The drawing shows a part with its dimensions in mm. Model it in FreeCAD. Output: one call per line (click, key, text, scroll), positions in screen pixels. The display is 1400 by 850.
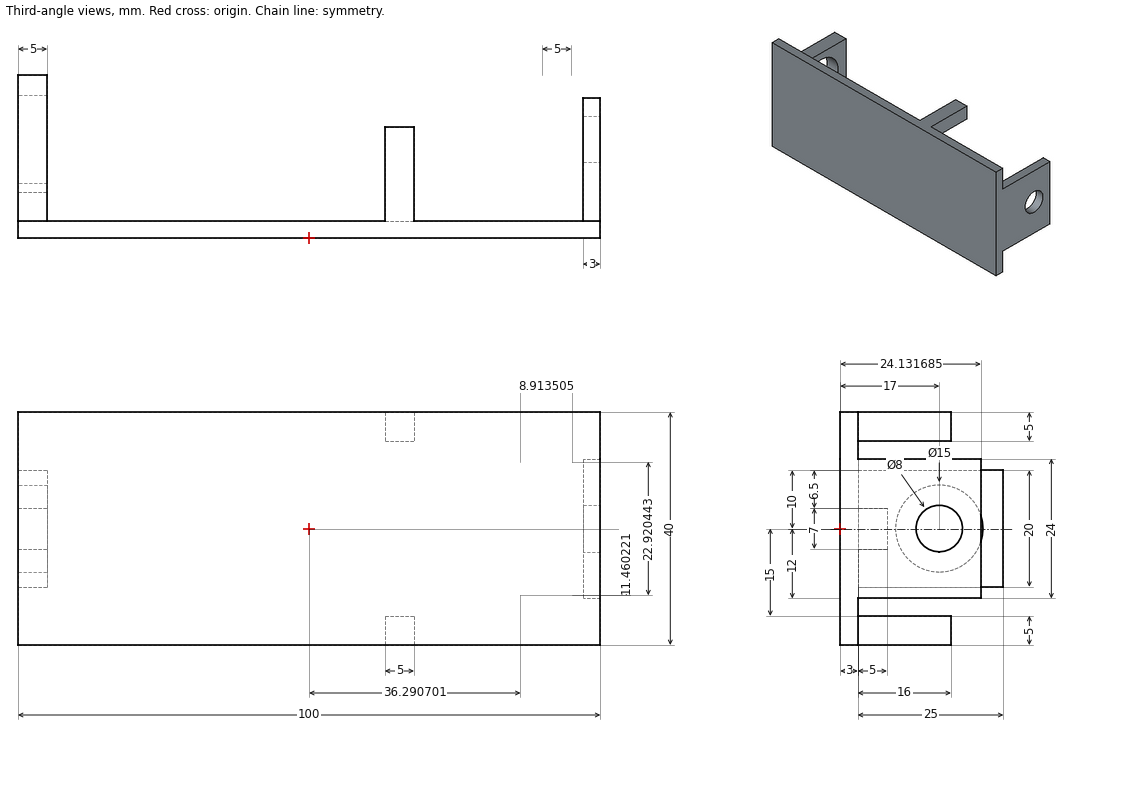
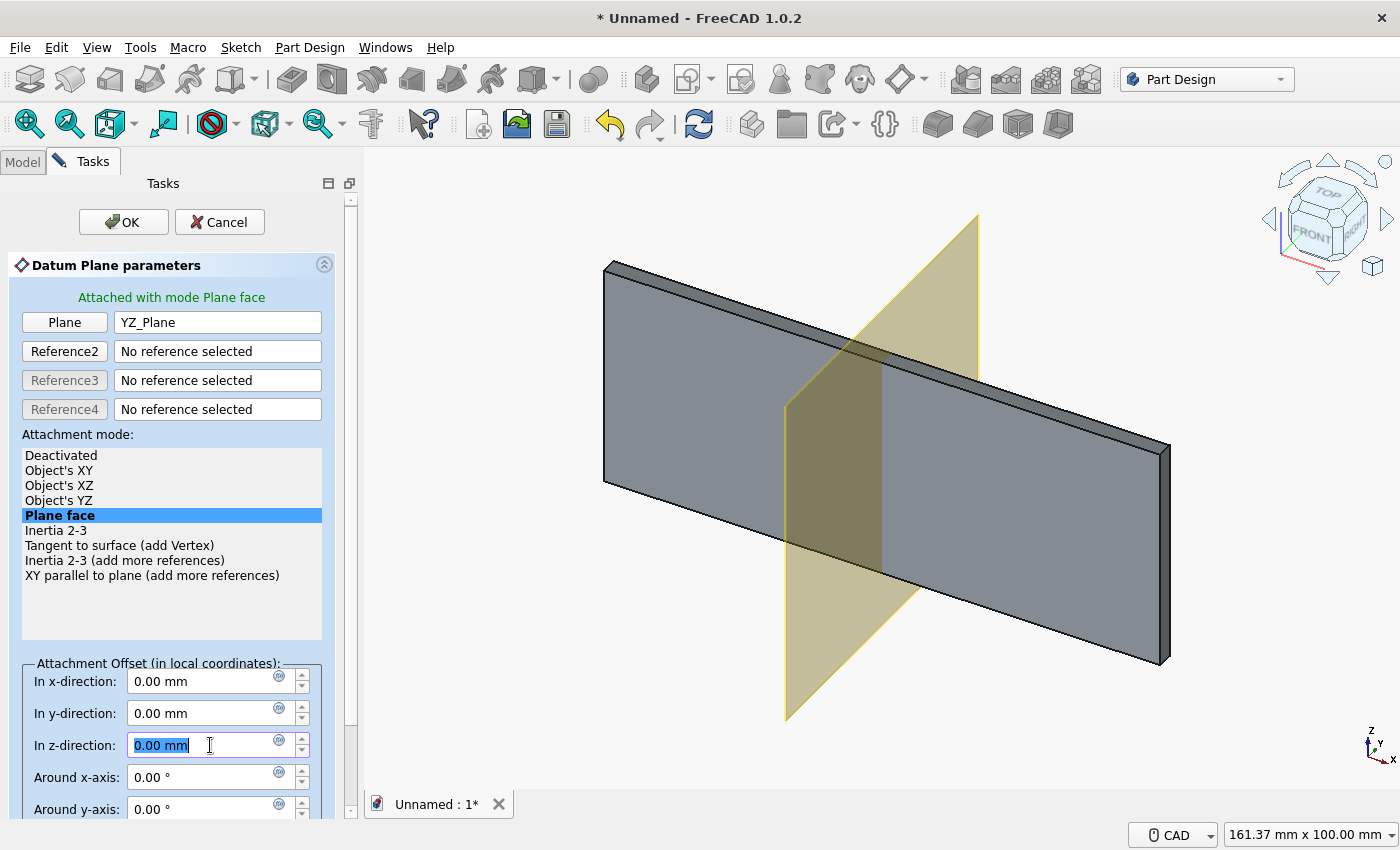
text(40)
key(Tab)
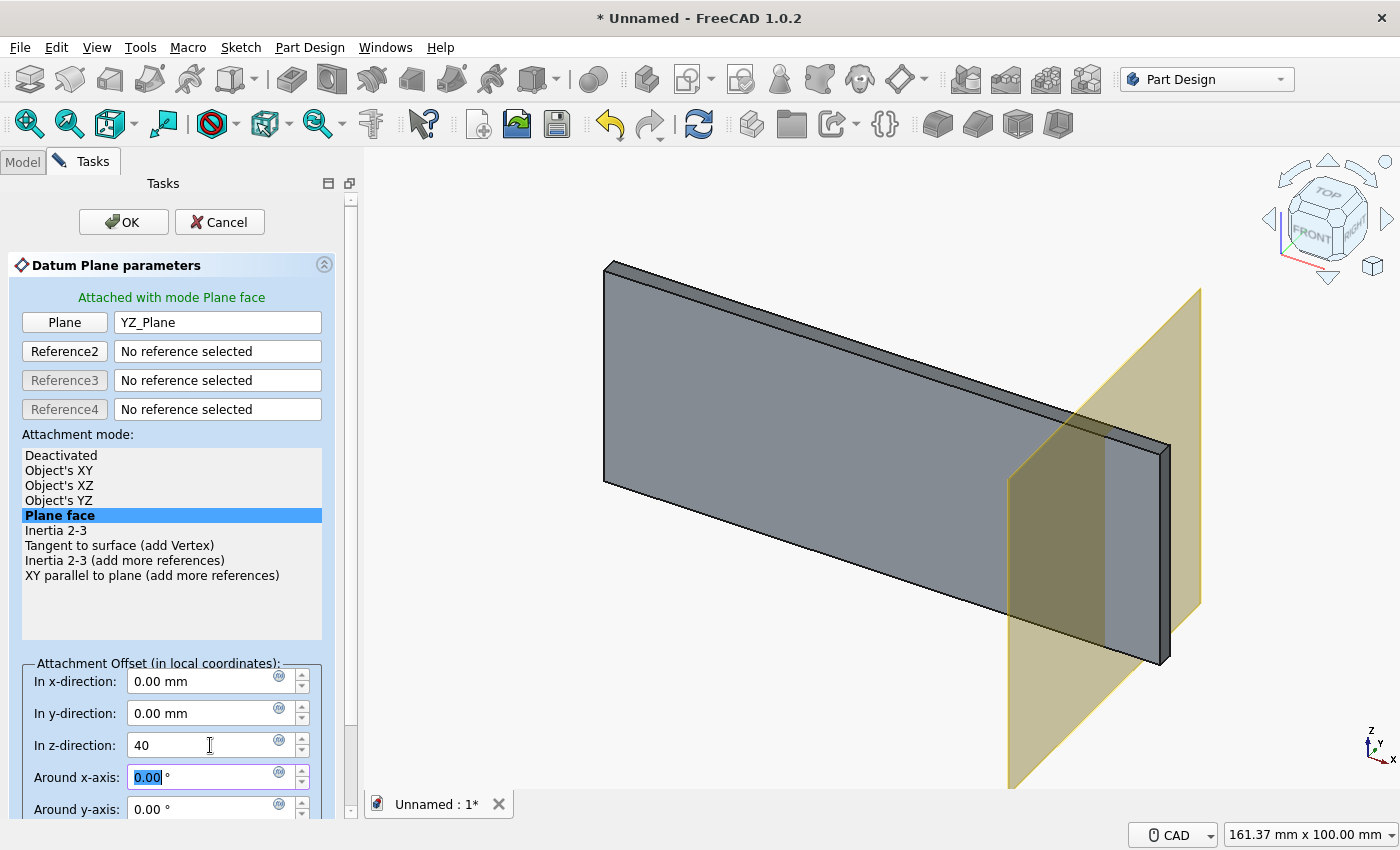
click(124, 222)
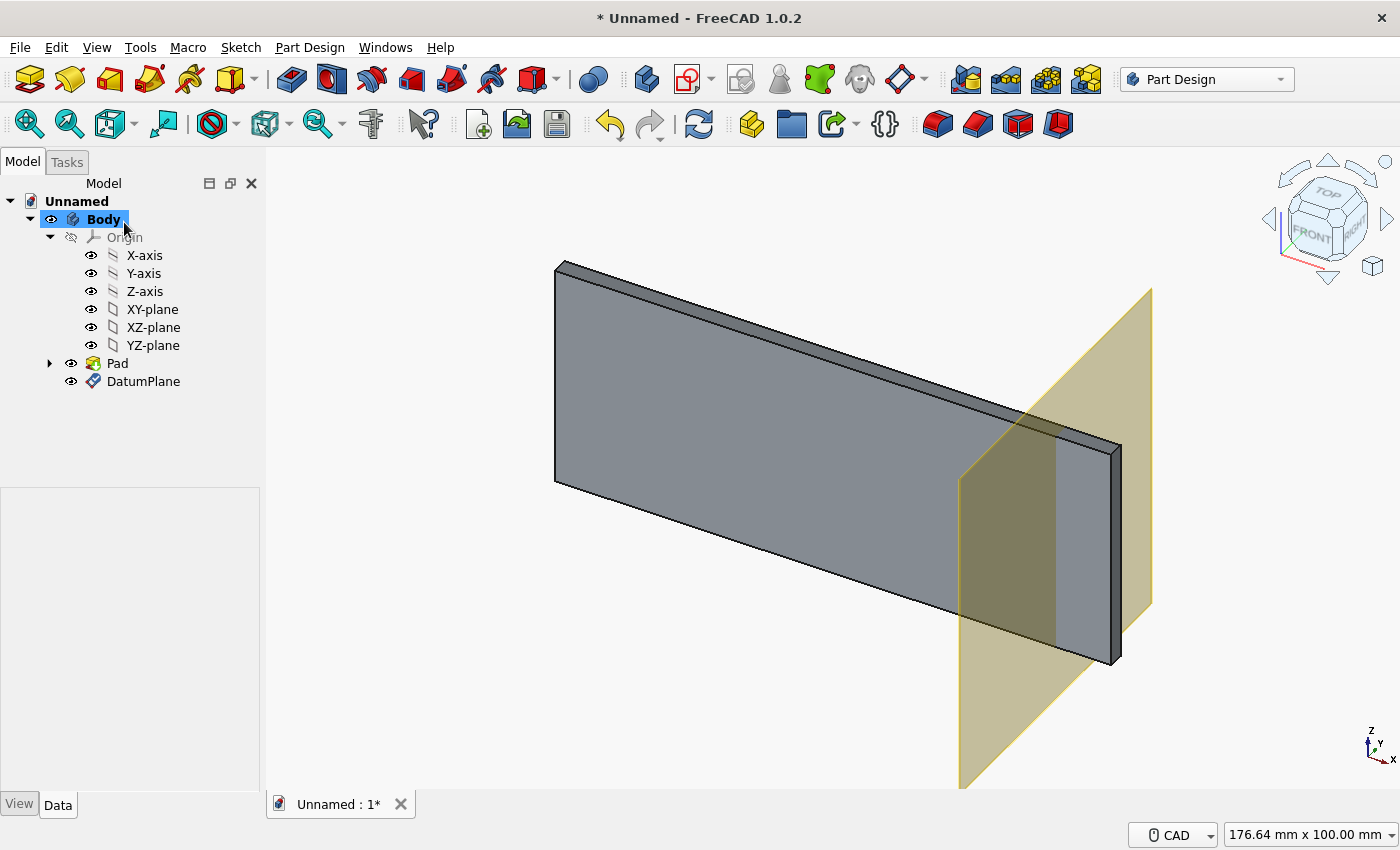
click(116, 381)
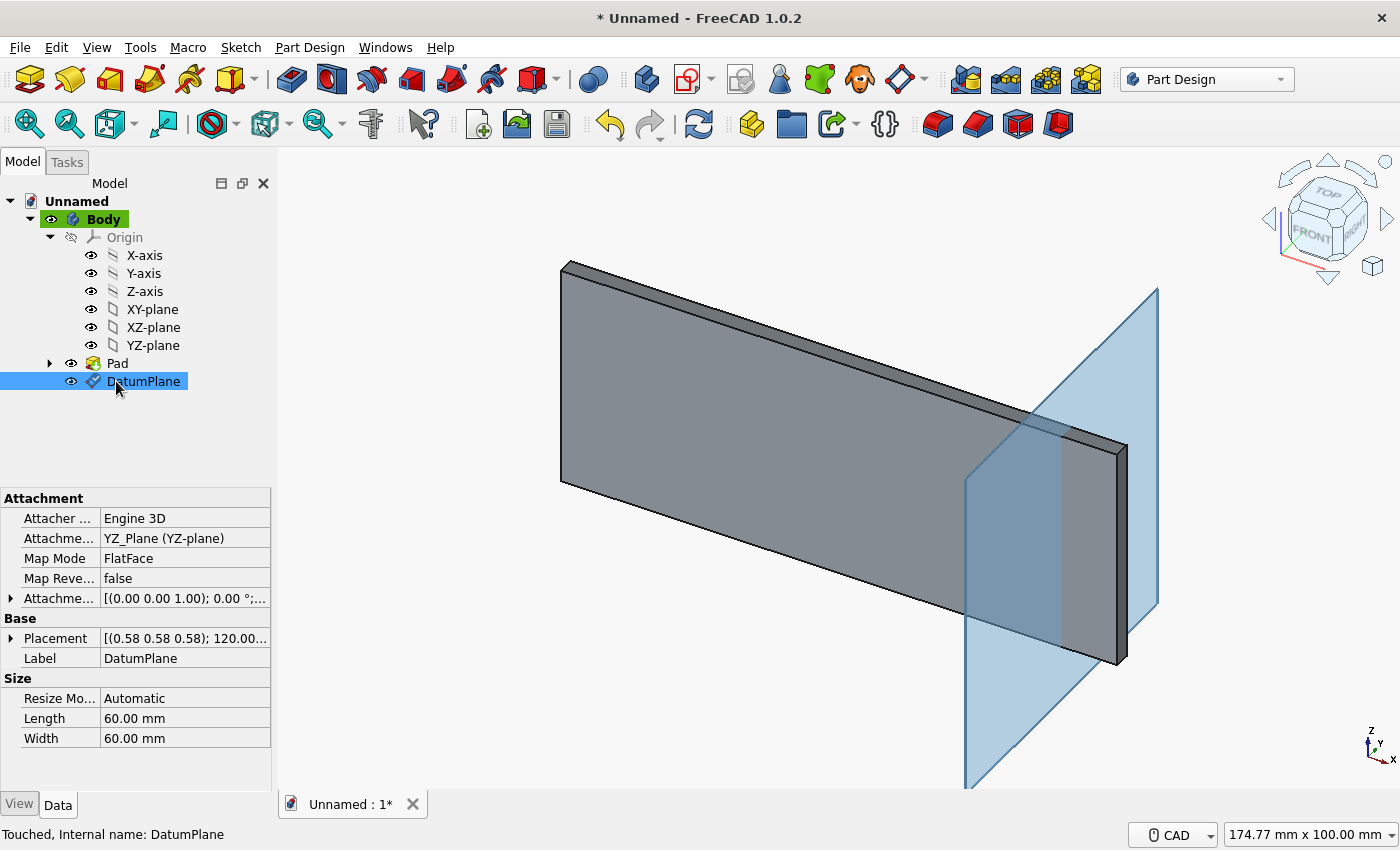
click(688, 80)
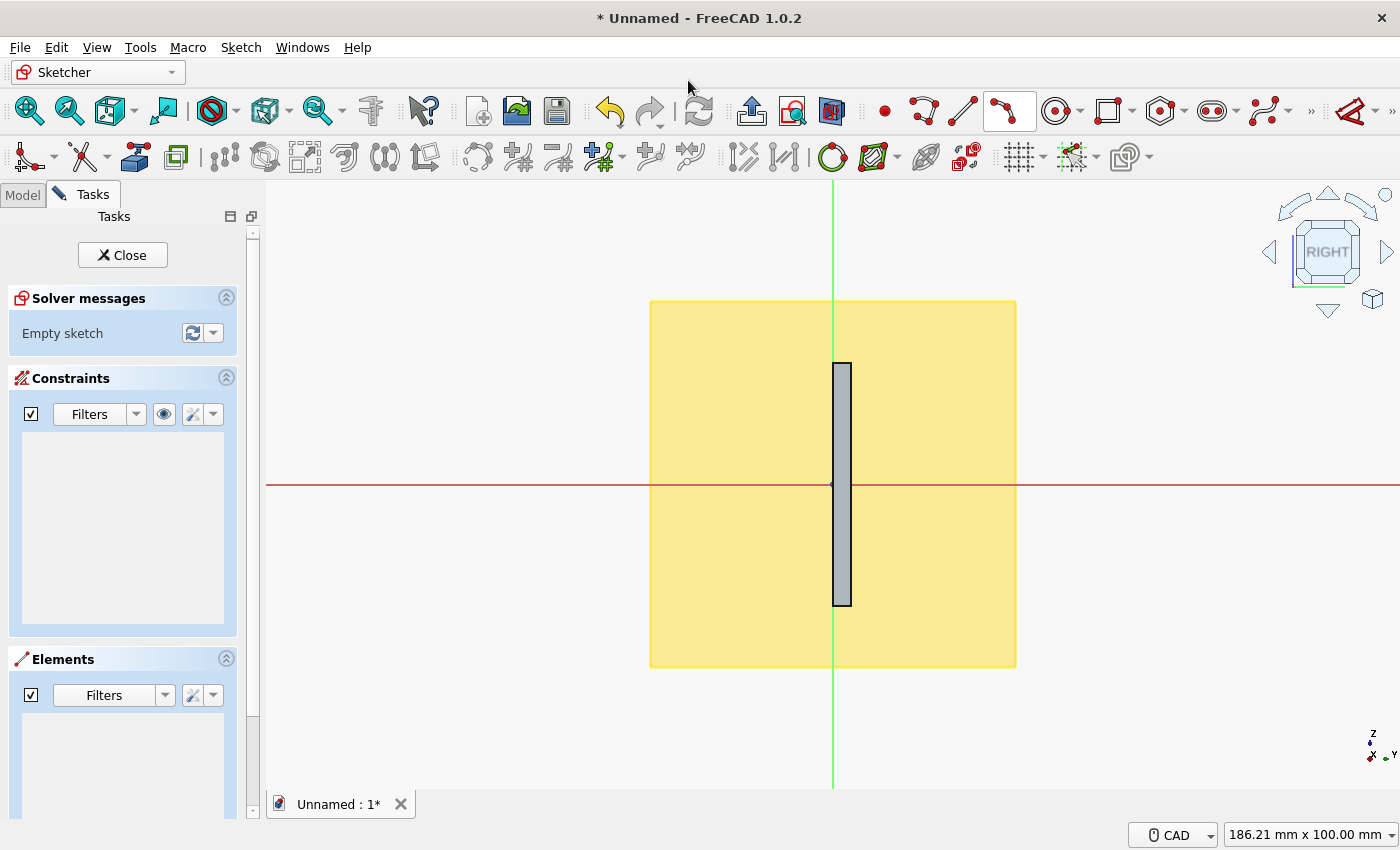
click(832, 112)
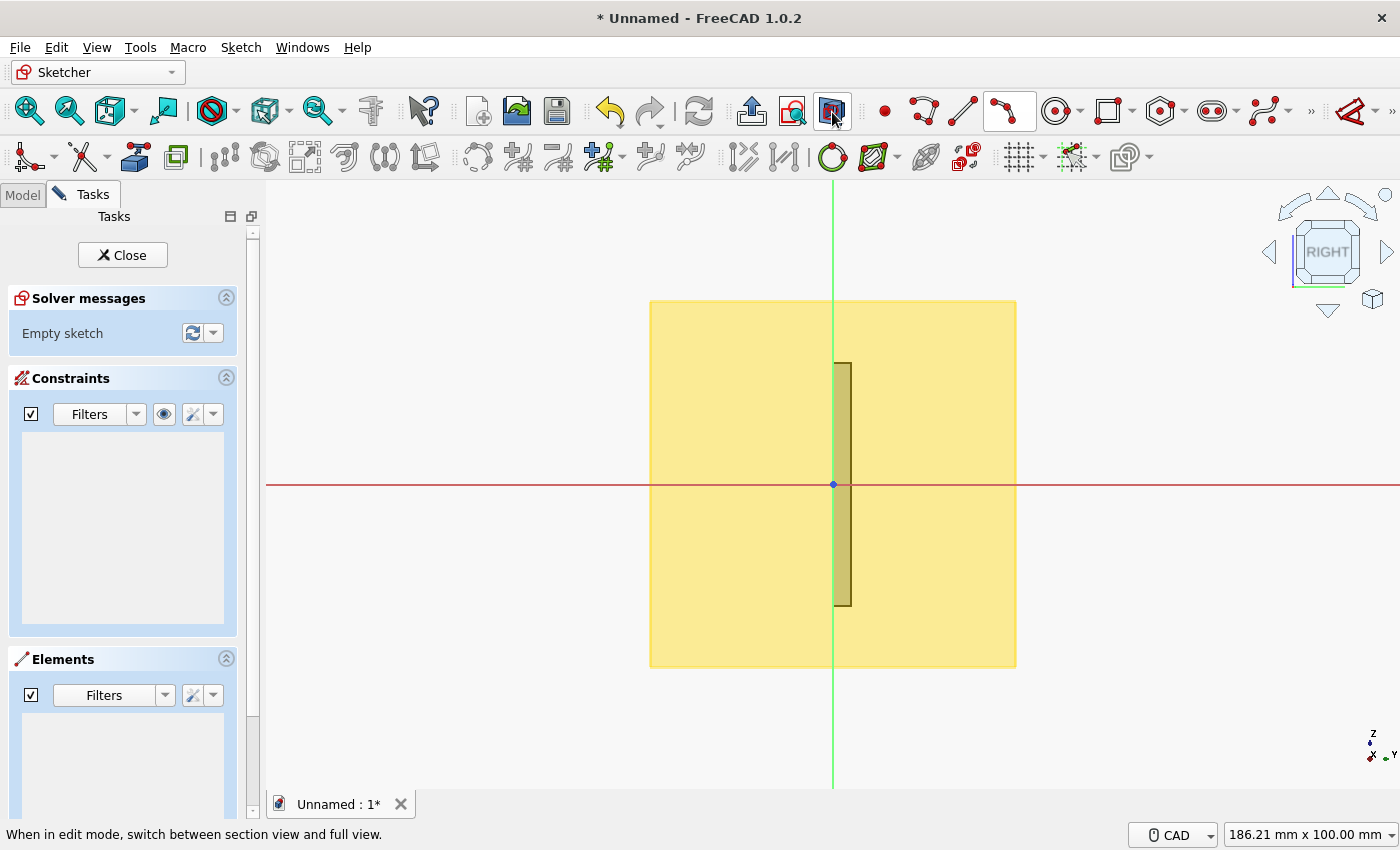
scroll(985, 484, up, 6)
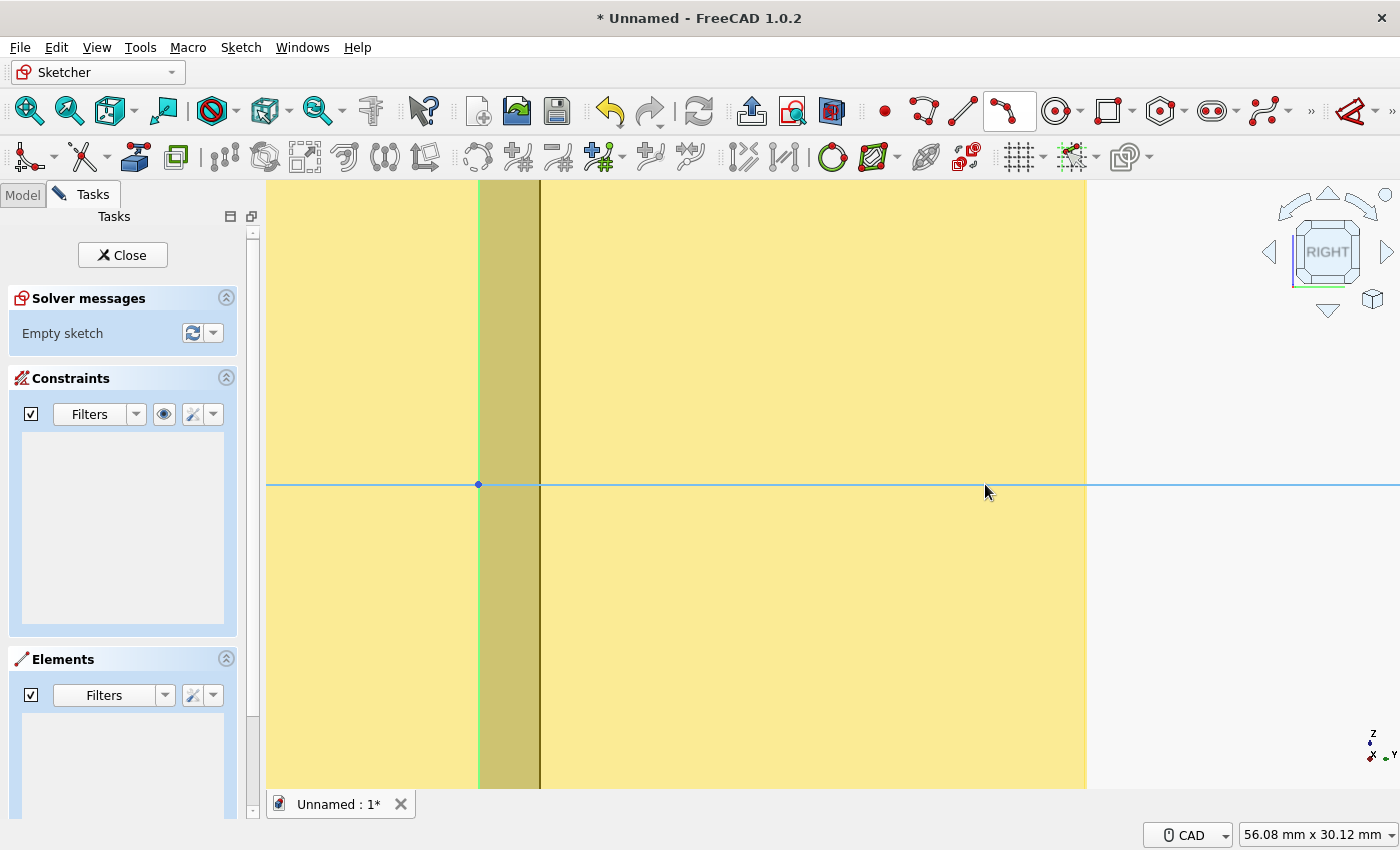
key(g)
key(r)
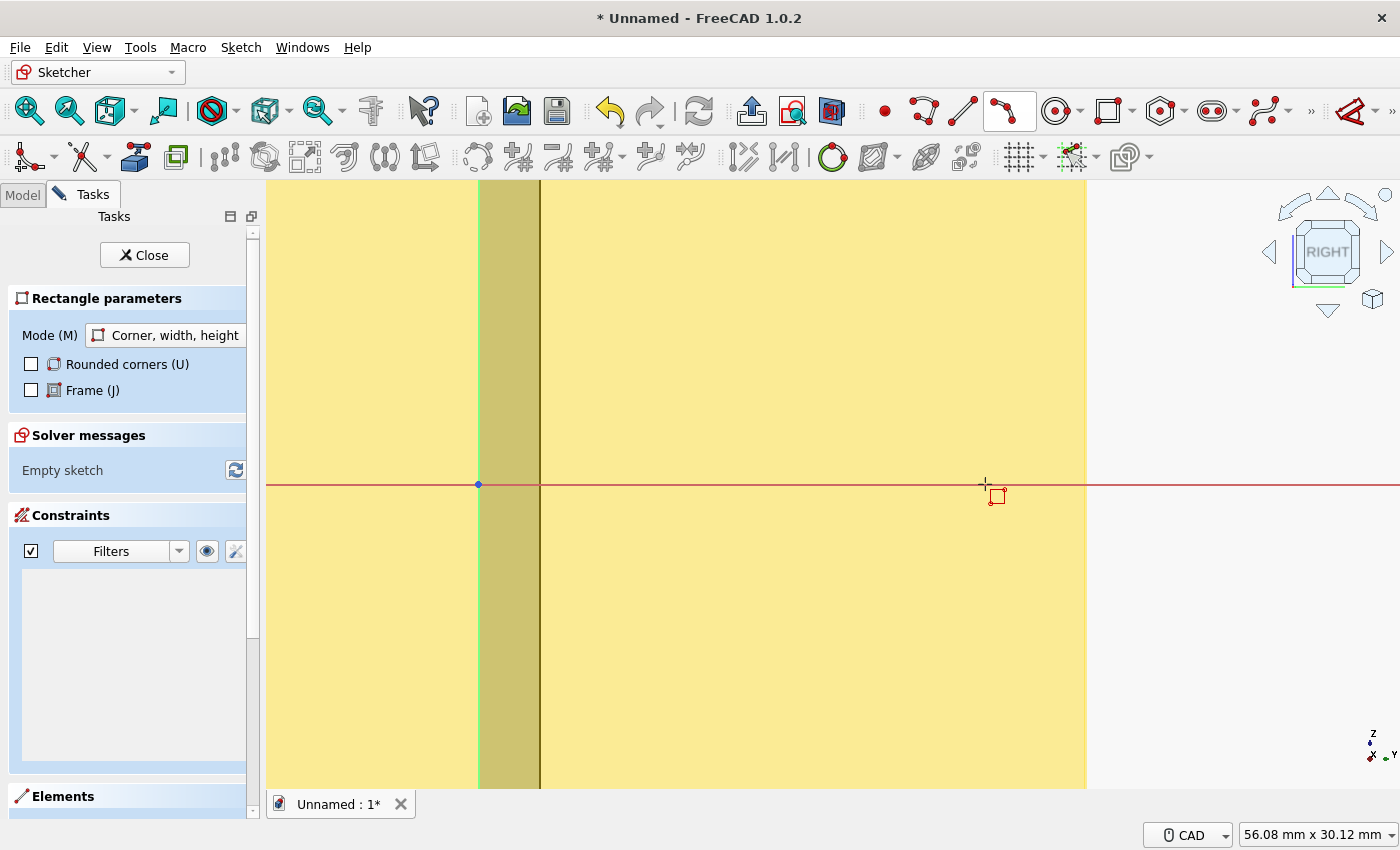
click(540, 282)
move(1045, 687)